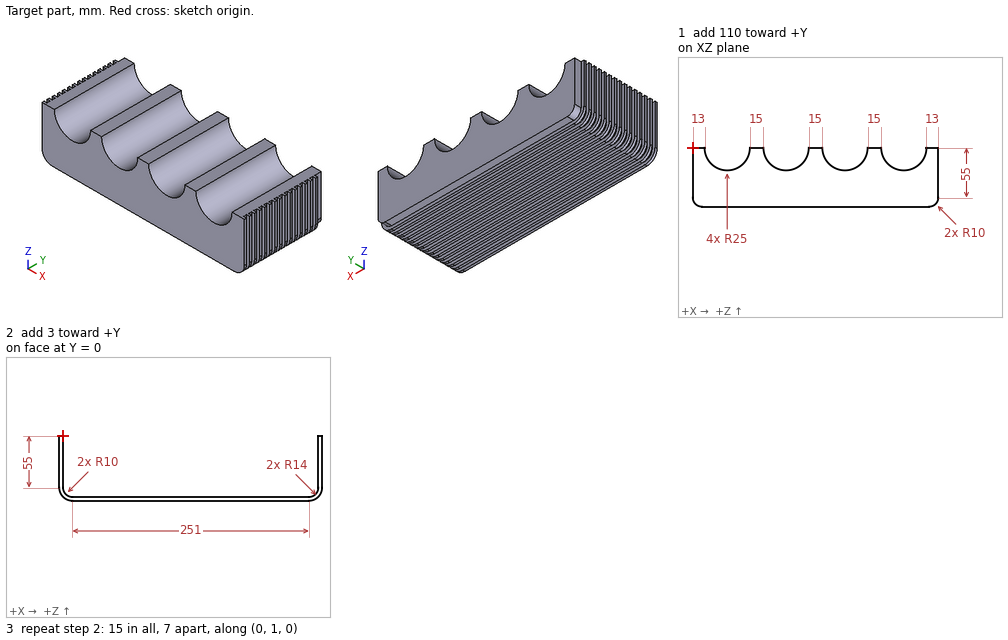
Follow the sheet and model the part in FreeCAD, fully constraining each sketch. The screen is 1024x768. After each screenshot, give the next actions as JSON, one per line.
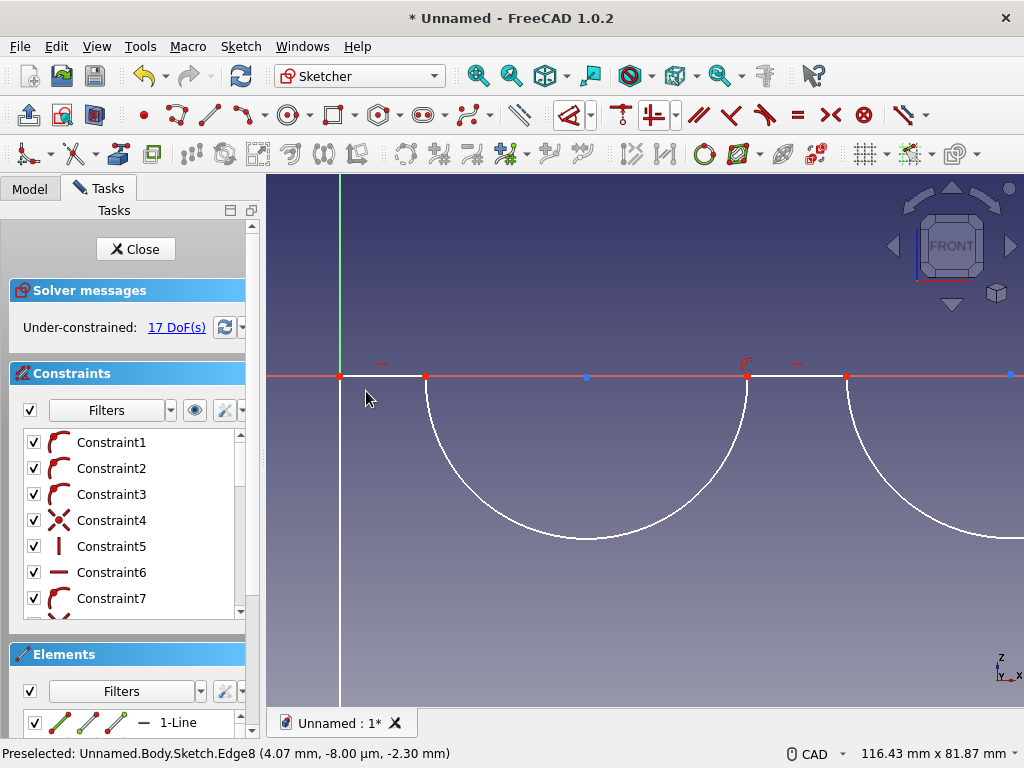
{"action": "scroll", "coordinate": [365, 392], "scroll_direction": "down", "scroll_amount": 7}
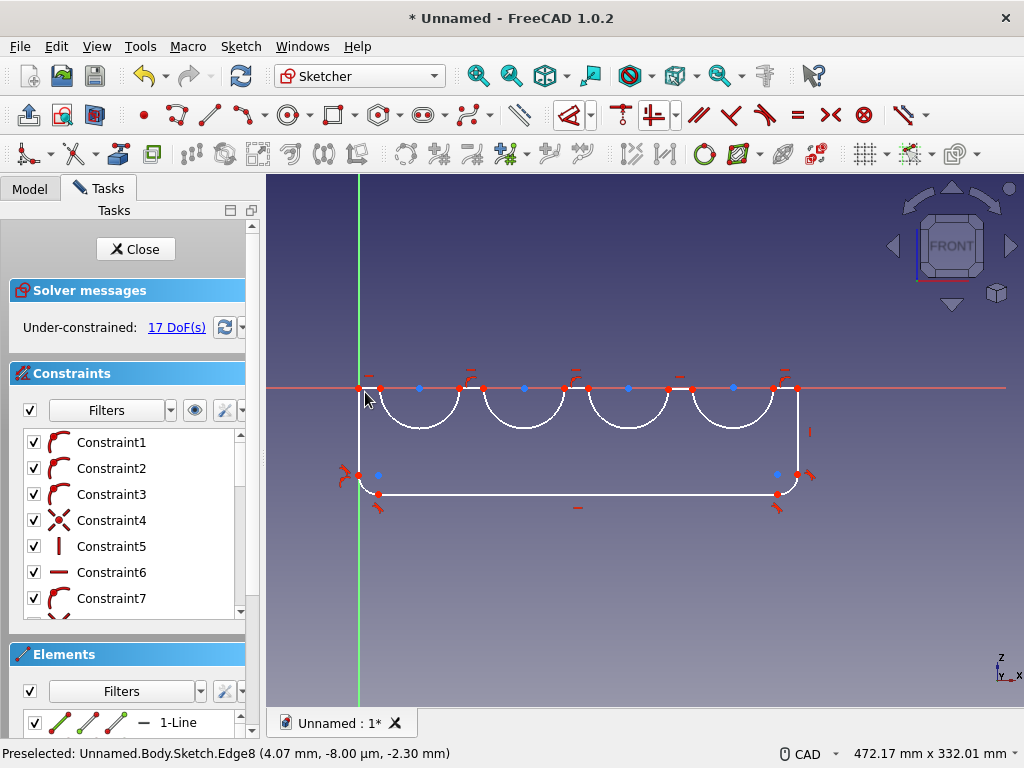
{"action": "left_click", "coordinate": [501, 421]}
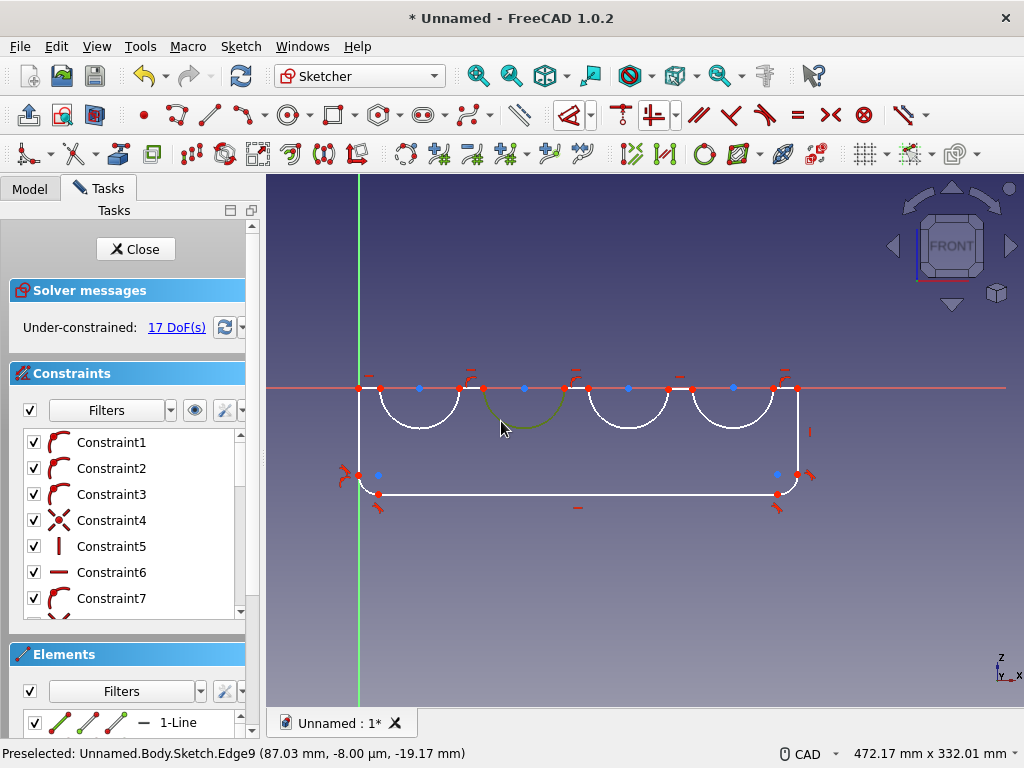
{"action": "left_click", "coordinate": [605, 421]}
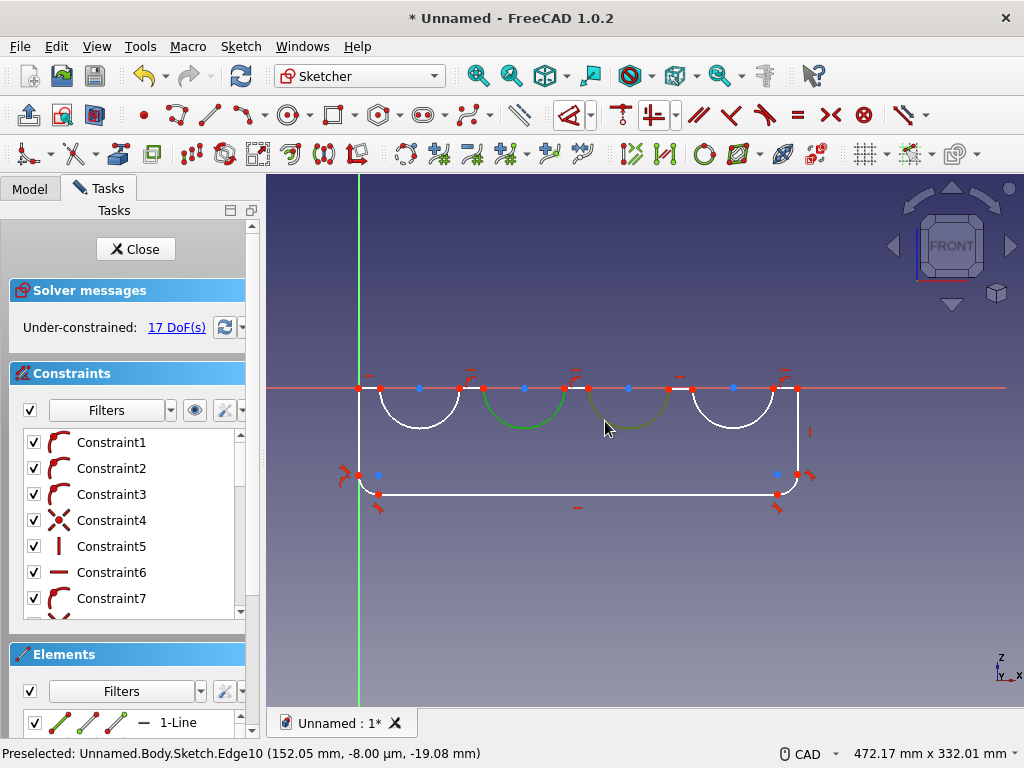
{"action": "left_click", "coordinate": [710, 421]}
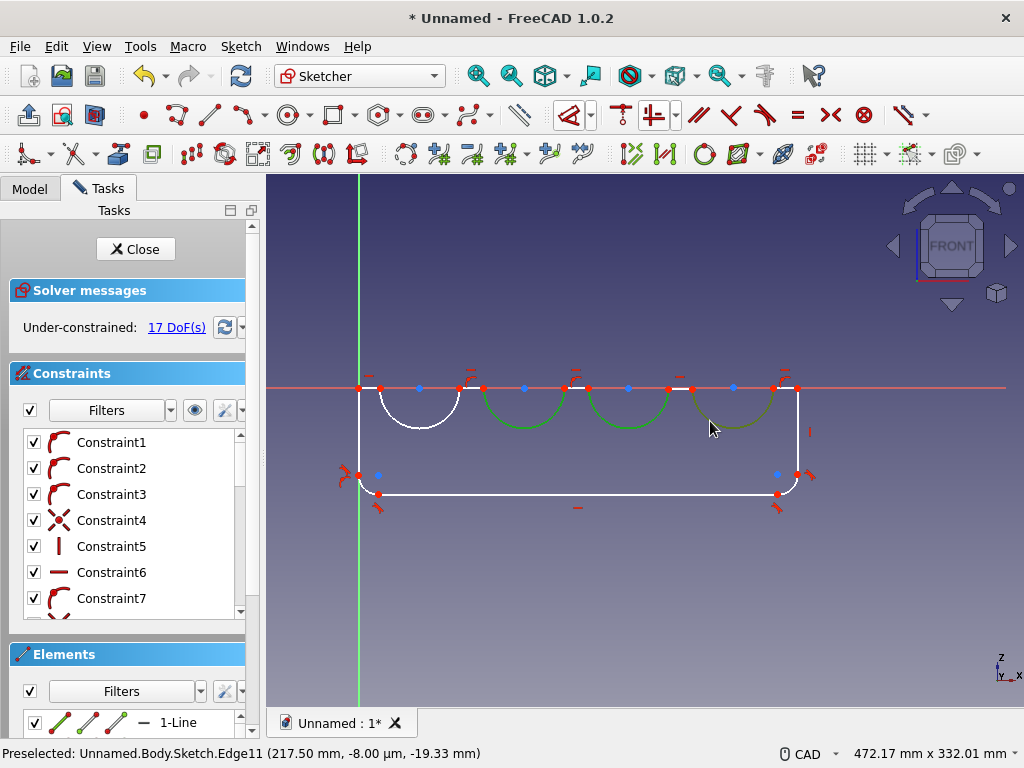
{"action": "left_click", "coordinate": [396, 421]}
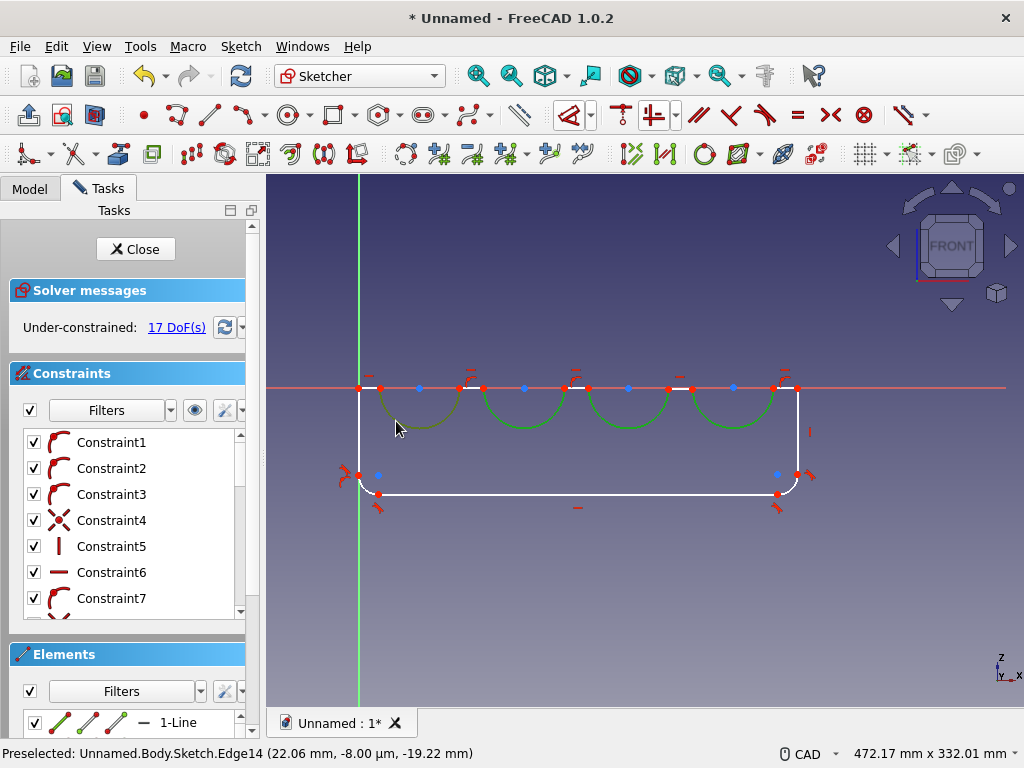
{"action": "left_click", "coordinate": [798, 116]}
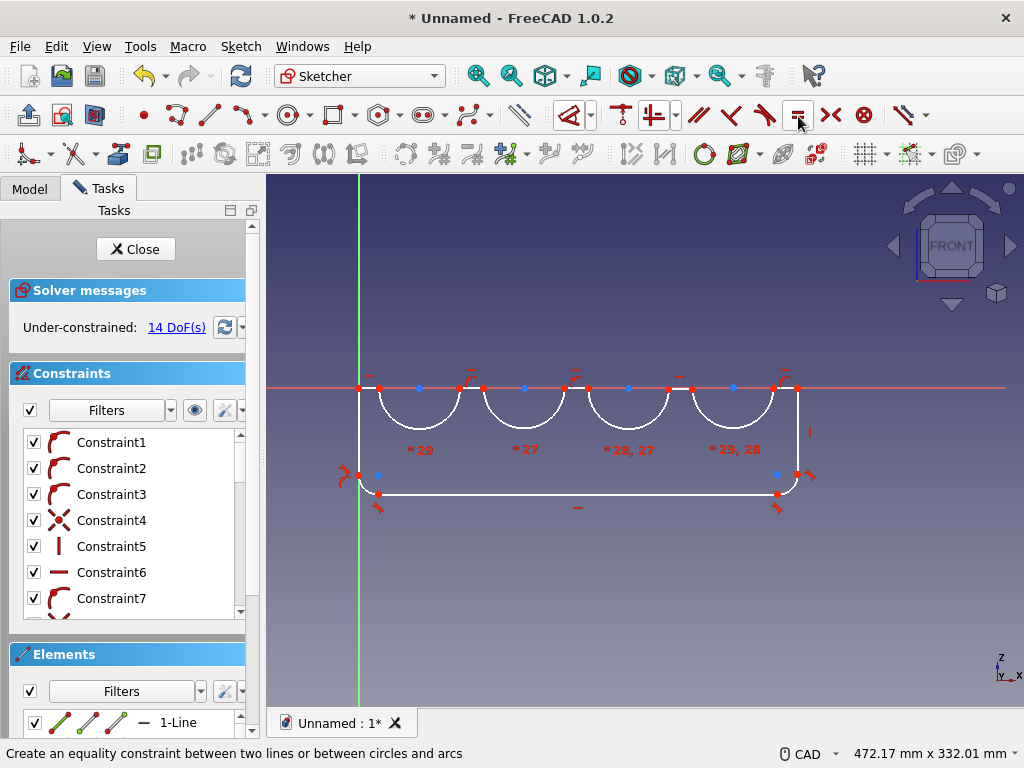
{"action": "scroll", "coordinate": [787, 492], "scroll_direction": "up", "scroll_amount": 3}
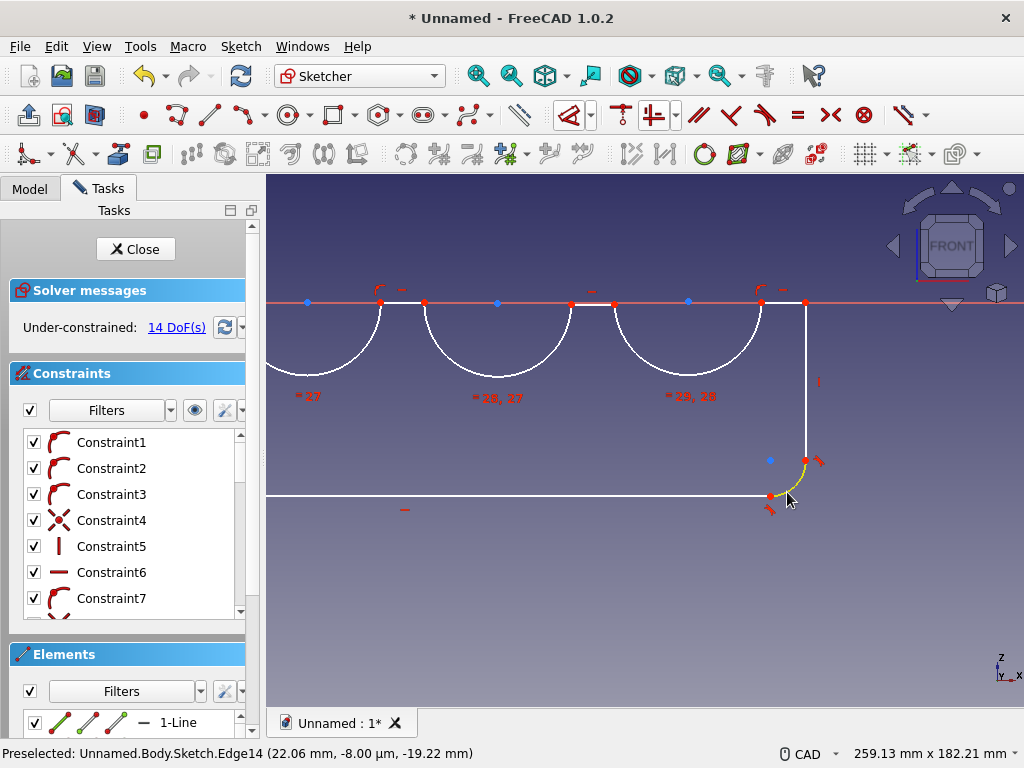
{"action": "left_click", "coordinate": [786, 492]}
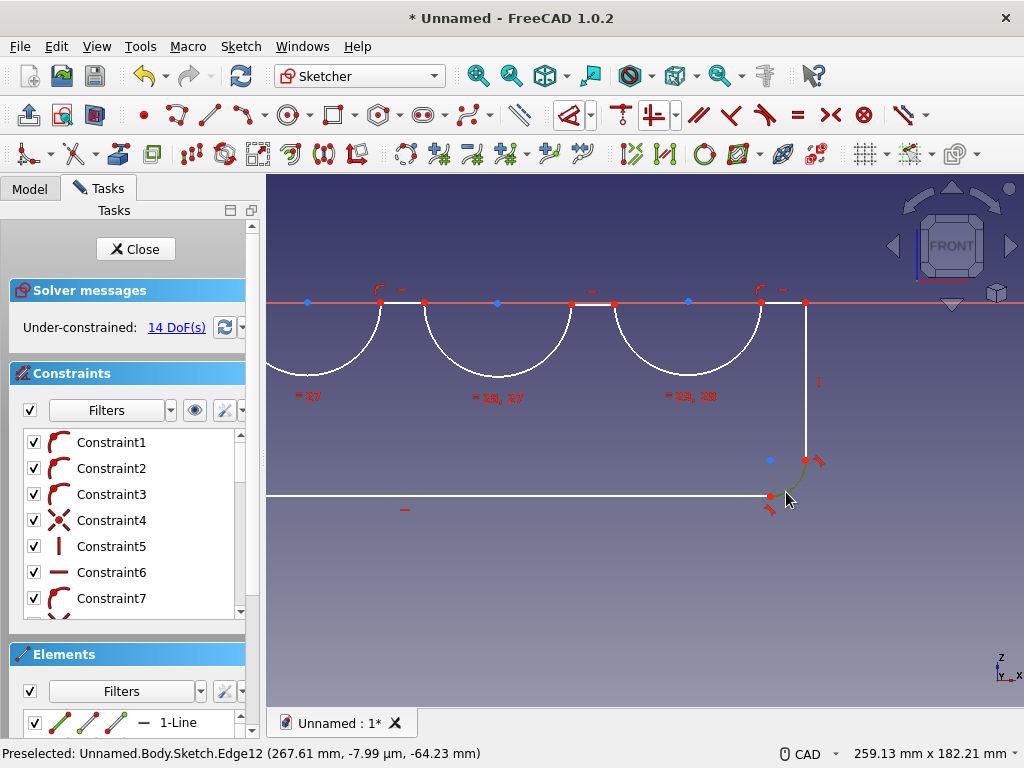
{"action": "scroll", "coordinate": [788, 492], "scroll_direction": "down", "scroll_amount": 3}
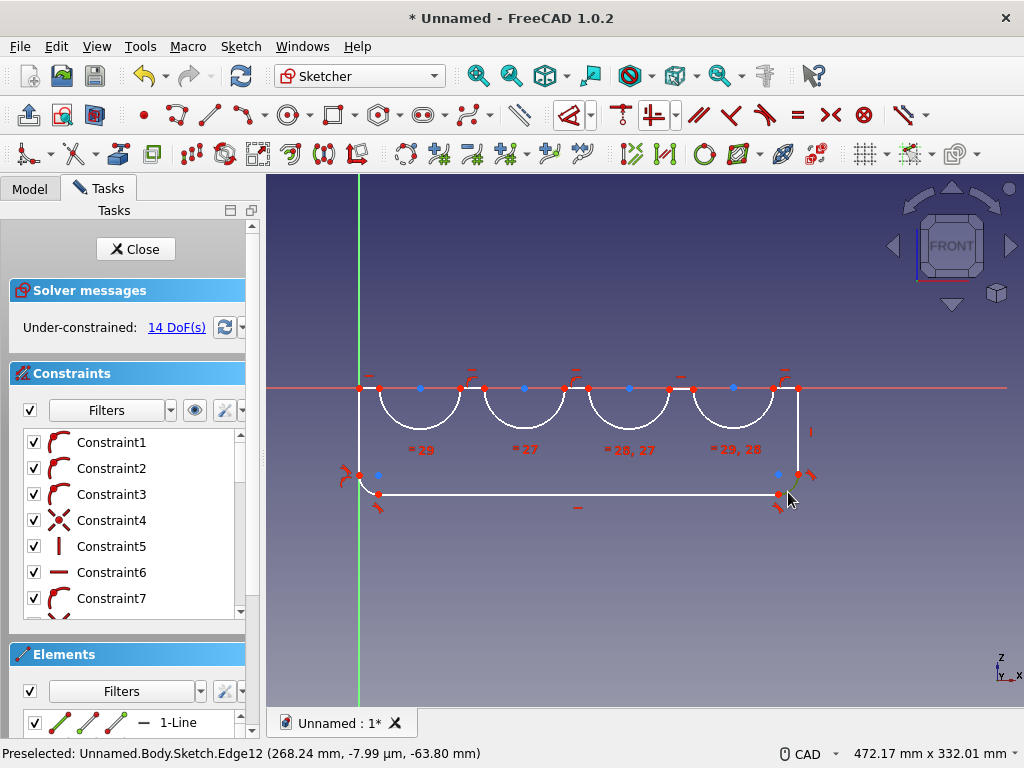
{"action": "scroll", "coordinate": [361, 484], "scroll_direction": "up", "scroll_amount": 3}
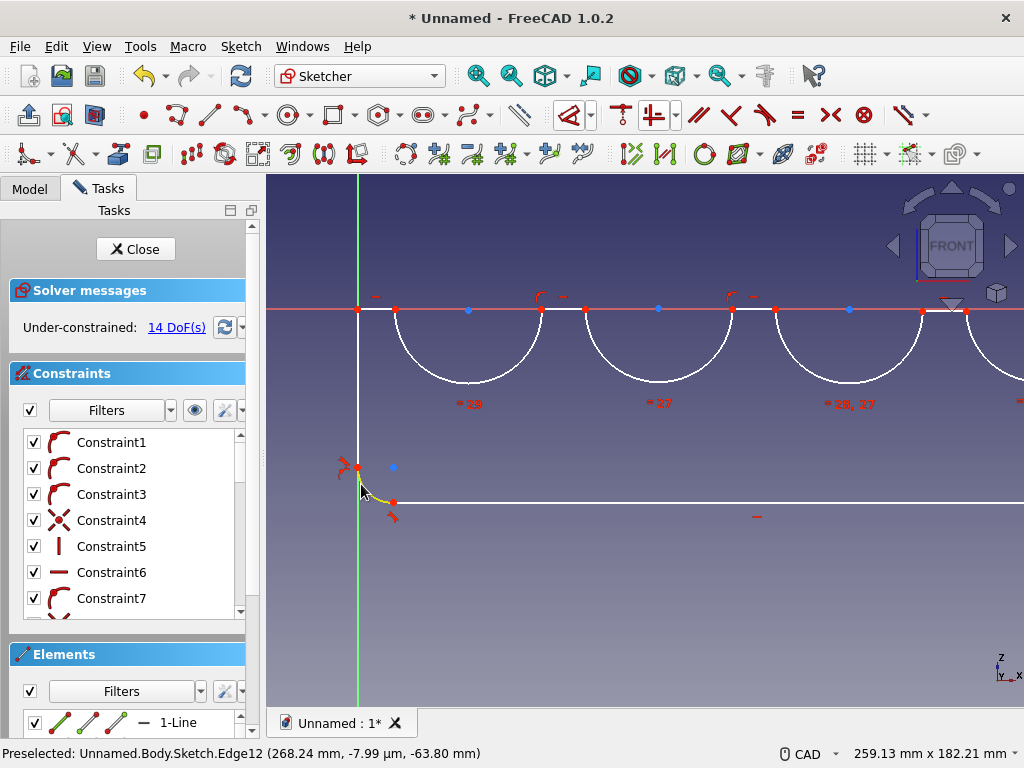
{"action": "left_click", "coordinate": [362, 484]}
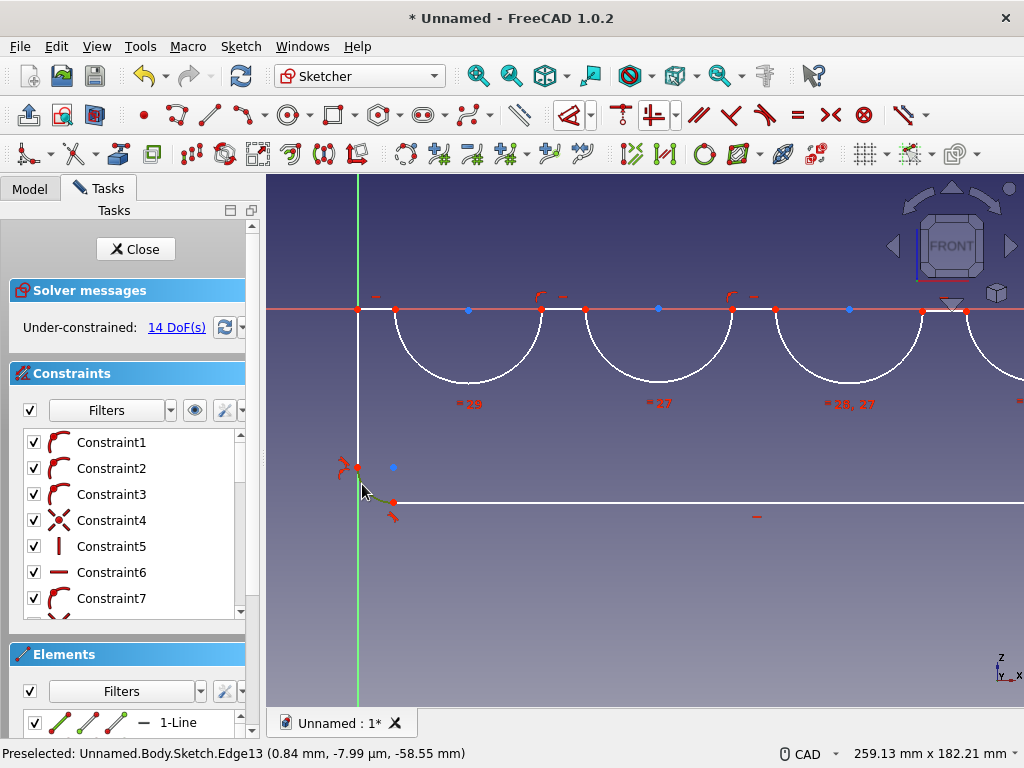
{"action": "left_click", "coordinate": [798, 116]}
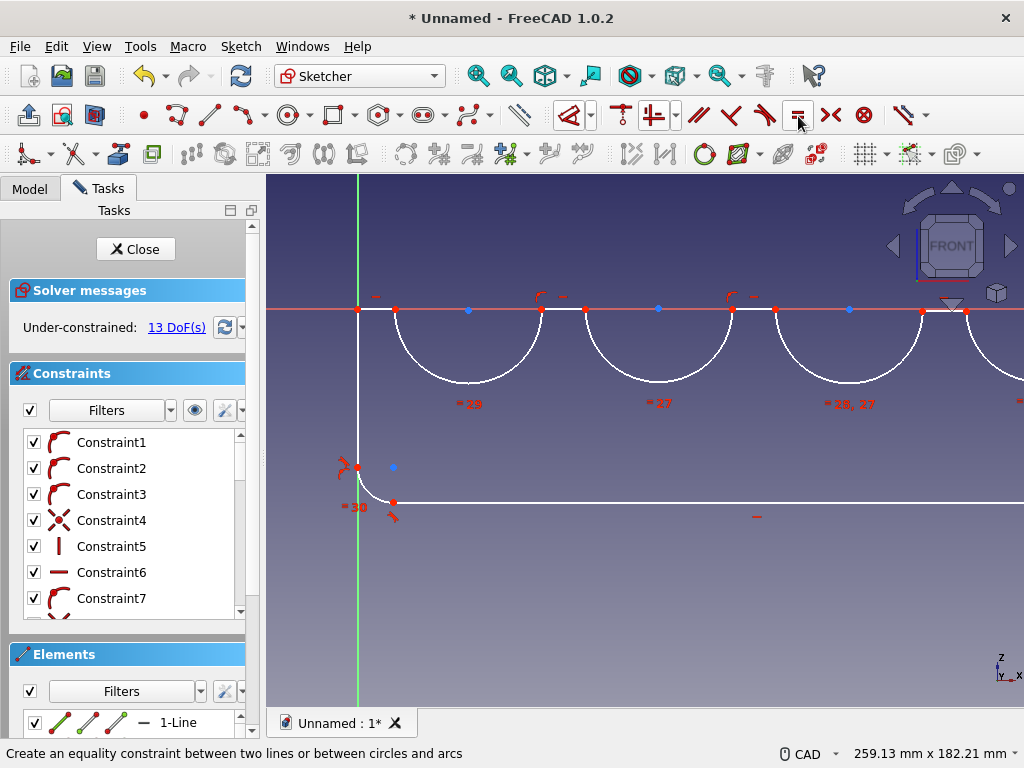
{"action": "left_click", "coordinate": [659, 309]}